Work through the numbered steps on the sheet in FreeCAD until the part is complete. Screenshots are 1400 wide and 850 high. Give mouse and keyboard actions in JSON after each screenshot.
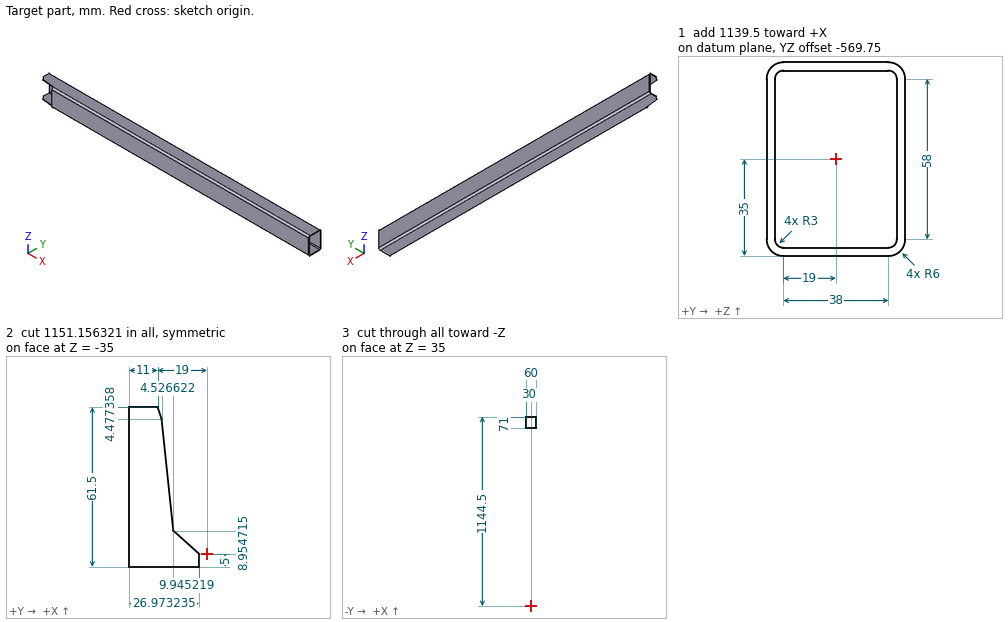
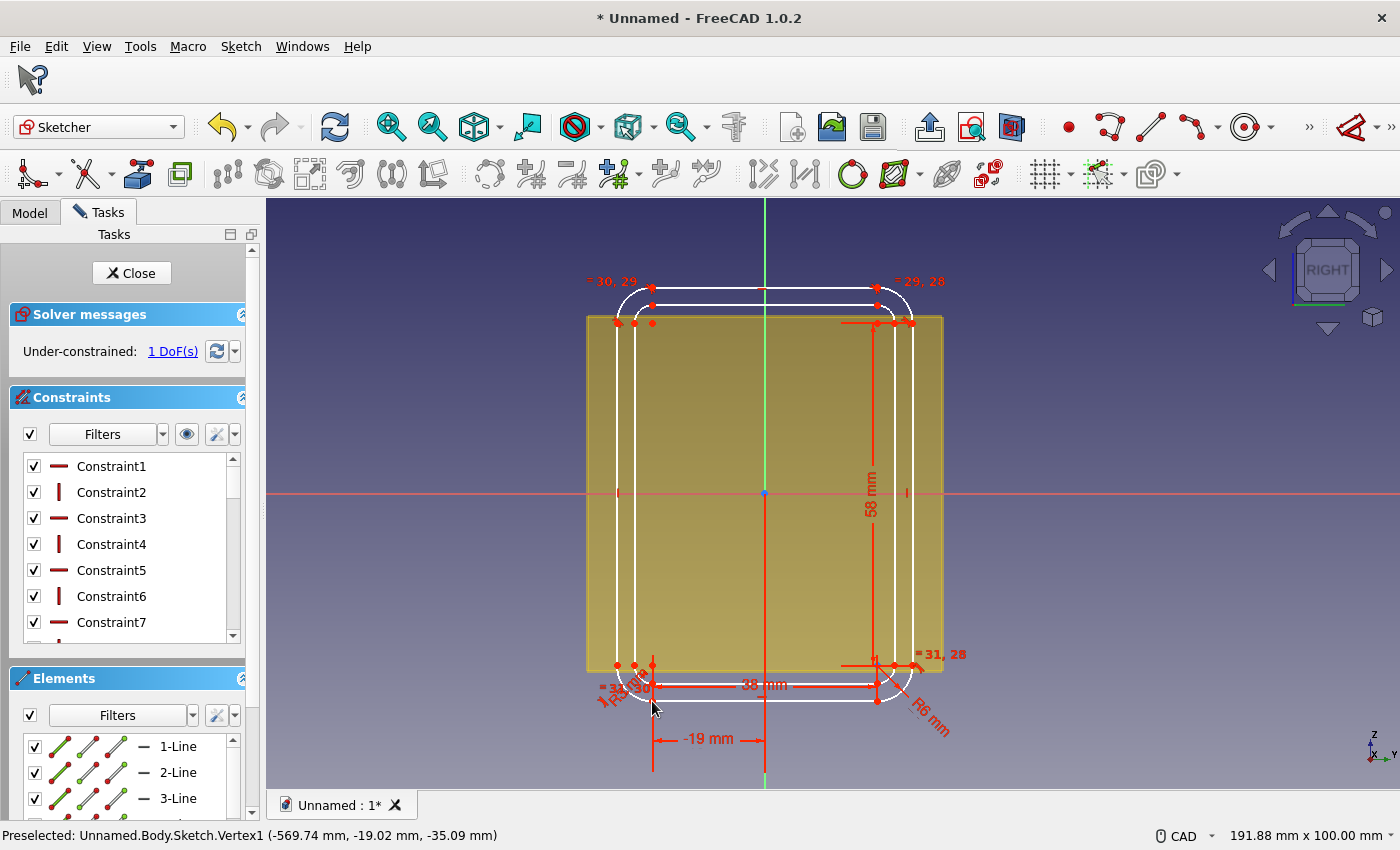
{"action": "left_click", "coordinate": [653, 701]}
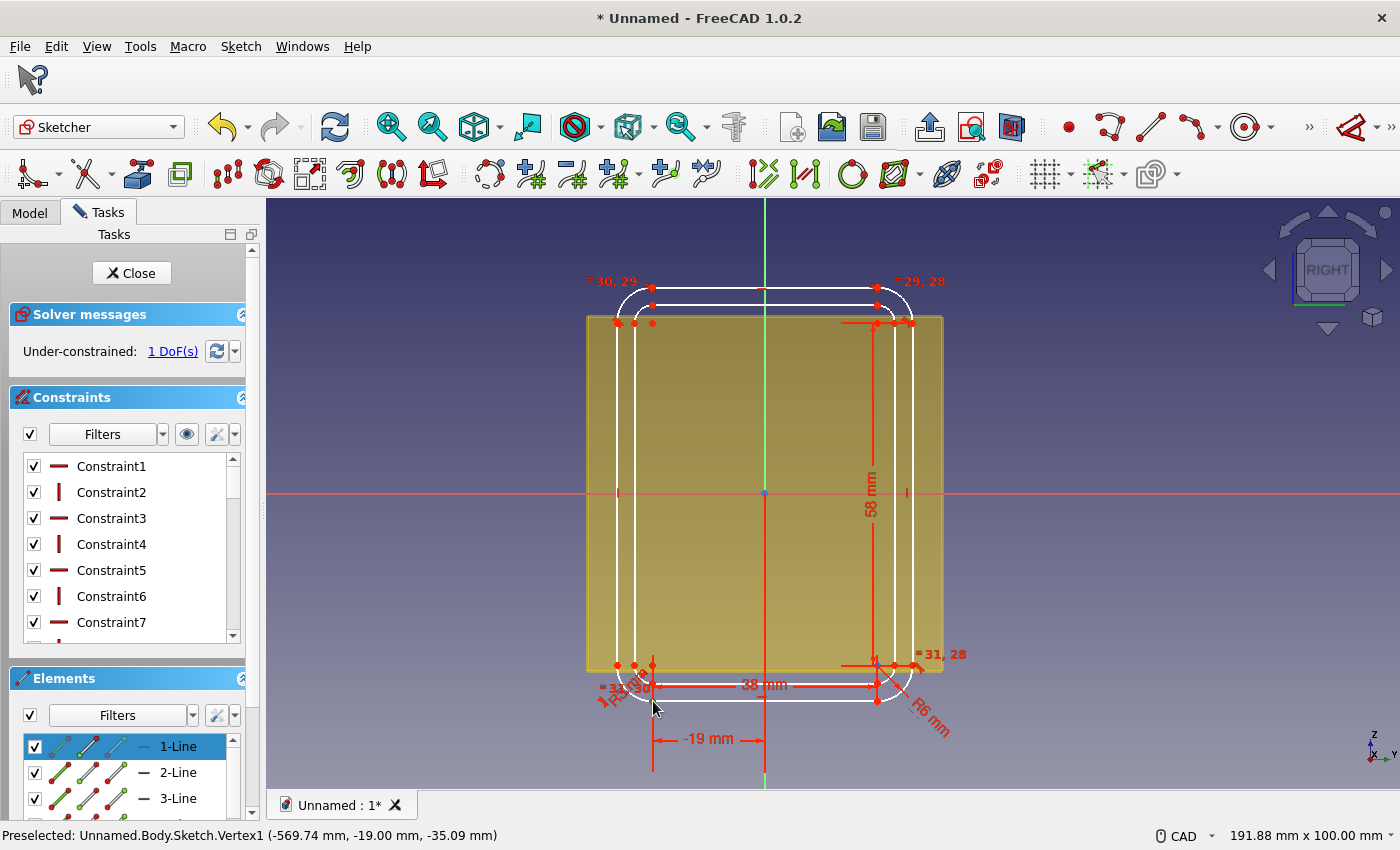
{"action": "left_click", "coordinate": [1376, 128]}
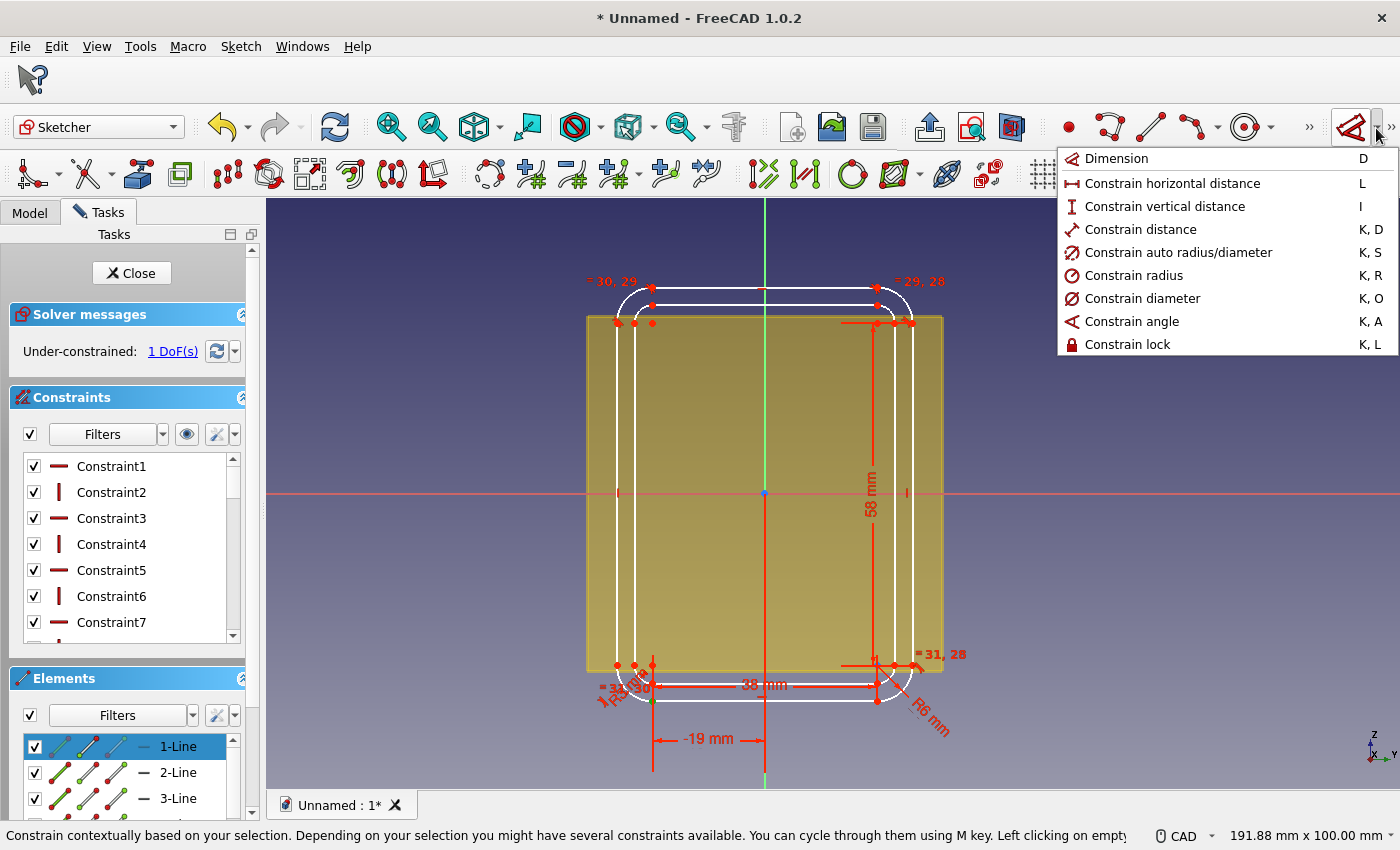
{"action": "left_click", "coordinate": [1228, 206]}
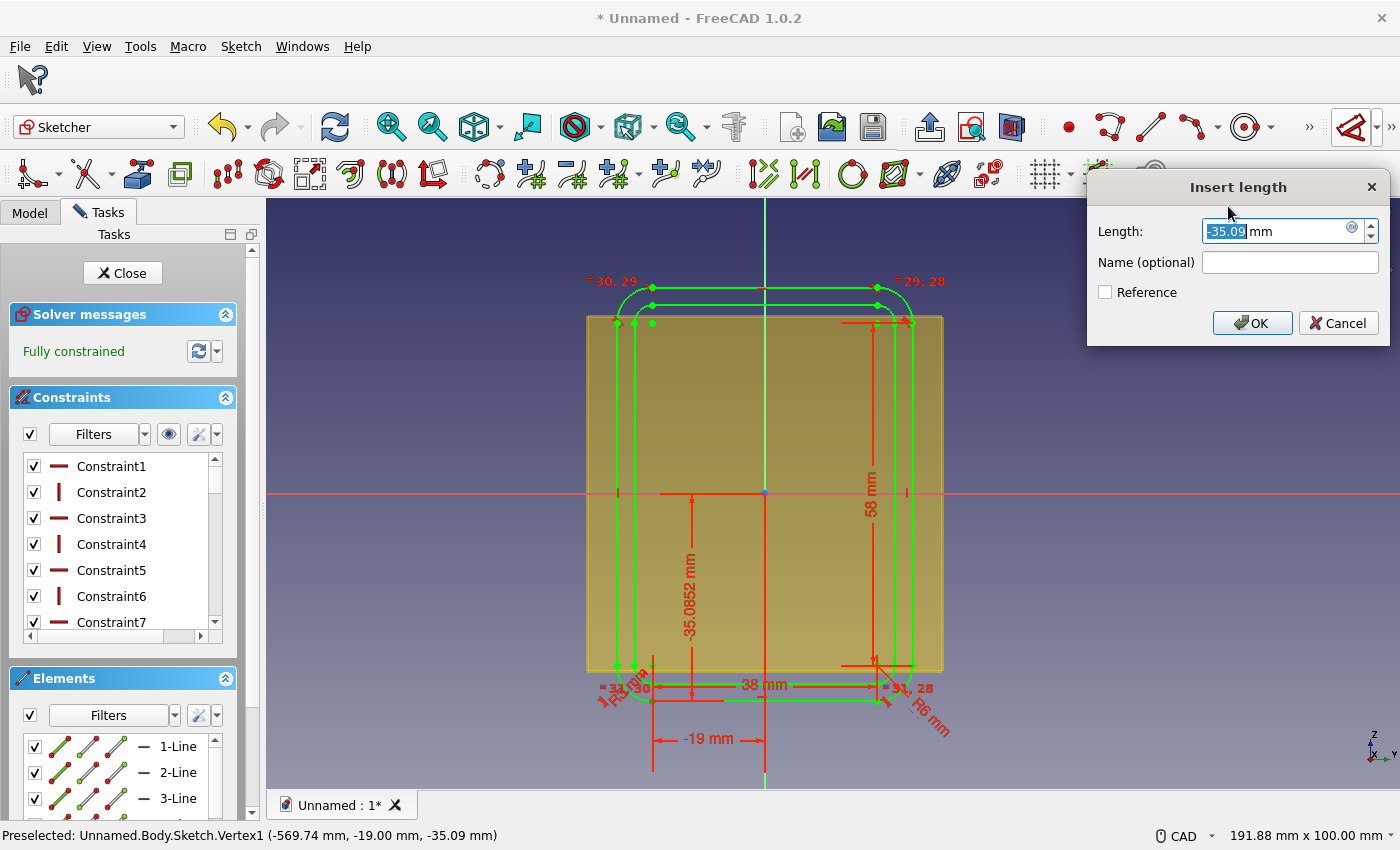
{"action": "type", "text": "-35"}
{"action": "key", "text": "Return"}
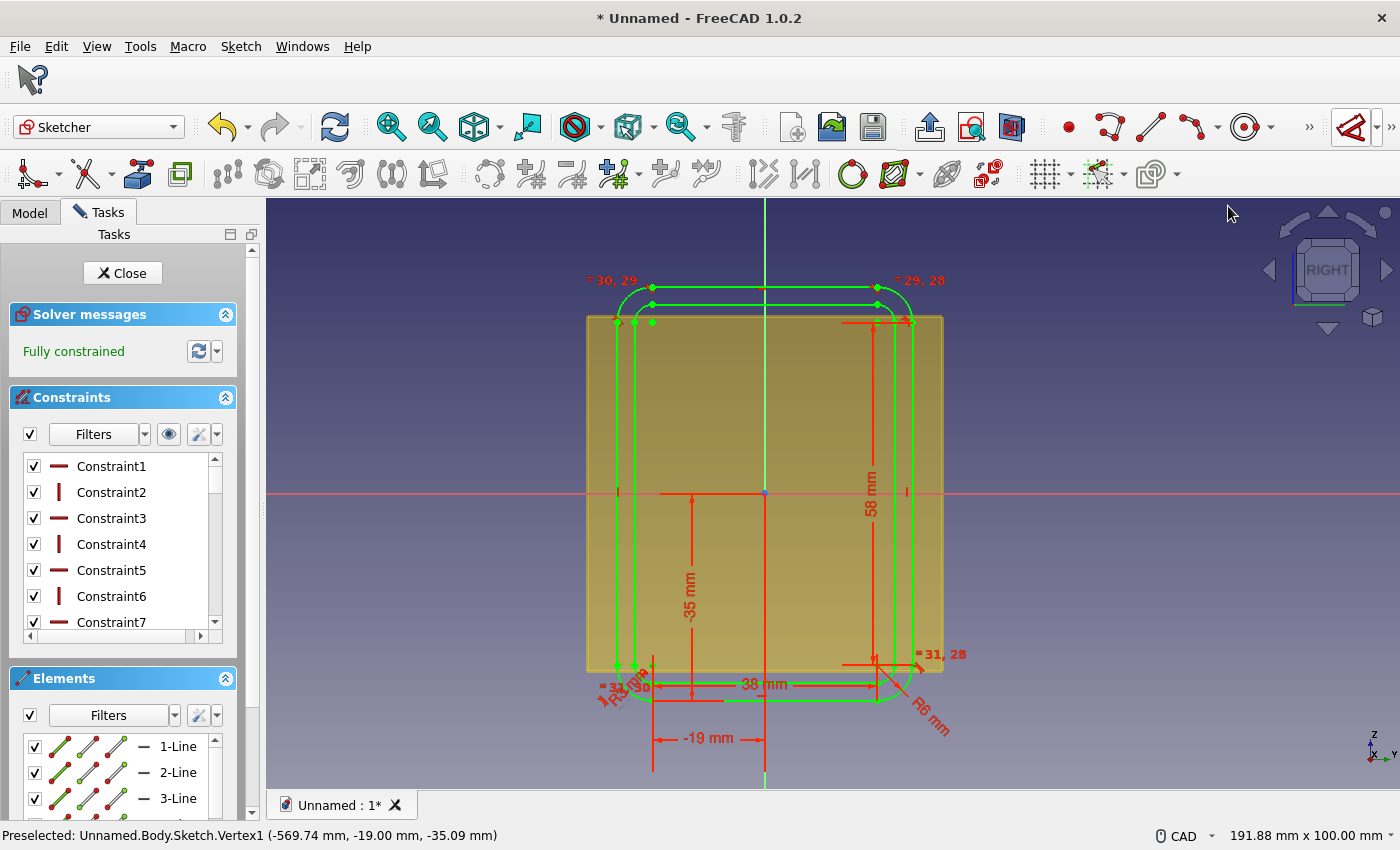
{"action": "left_click", "coordinate": [123, 273]}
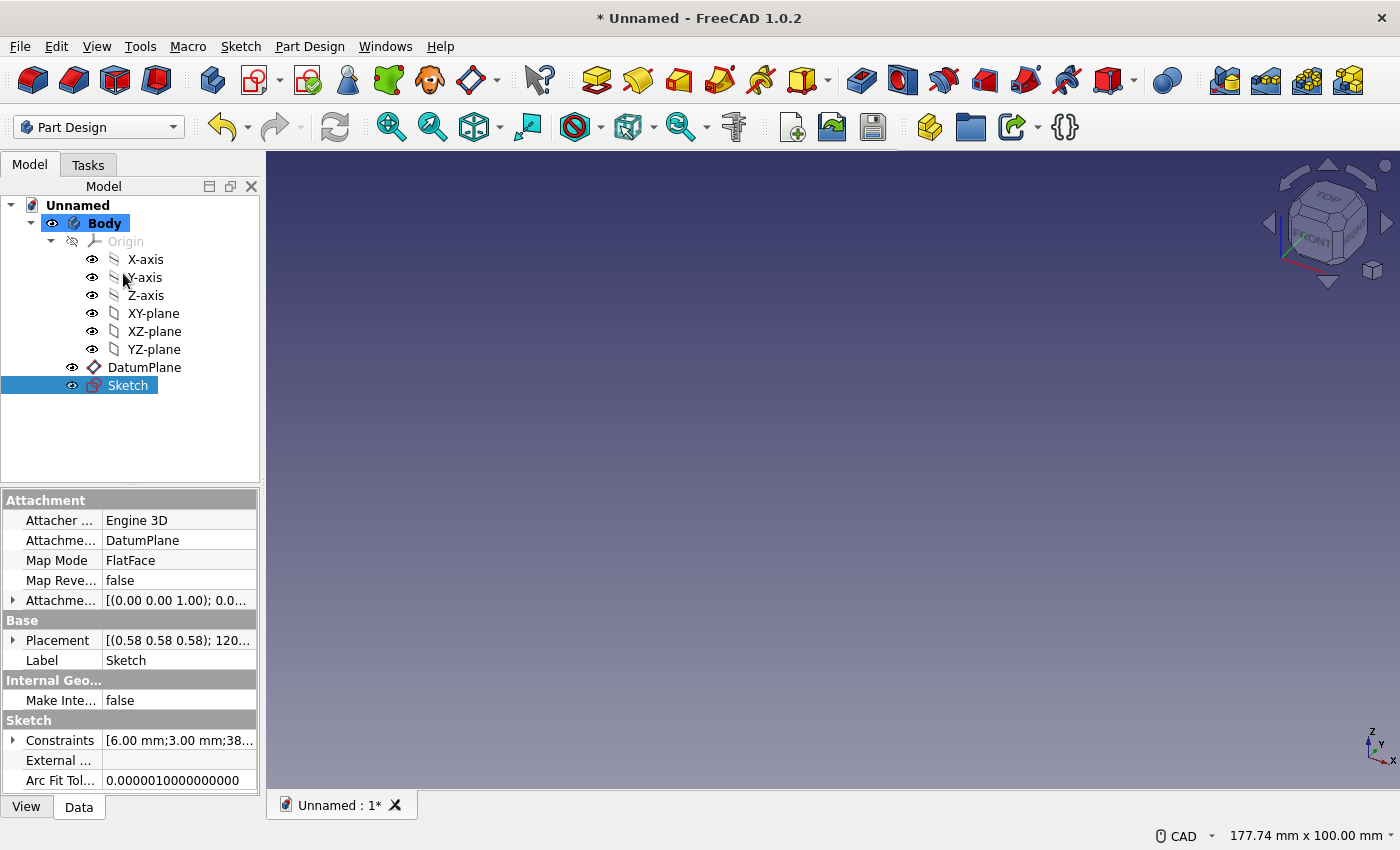
{"action": "left_click", "coordinate": [597, 80]}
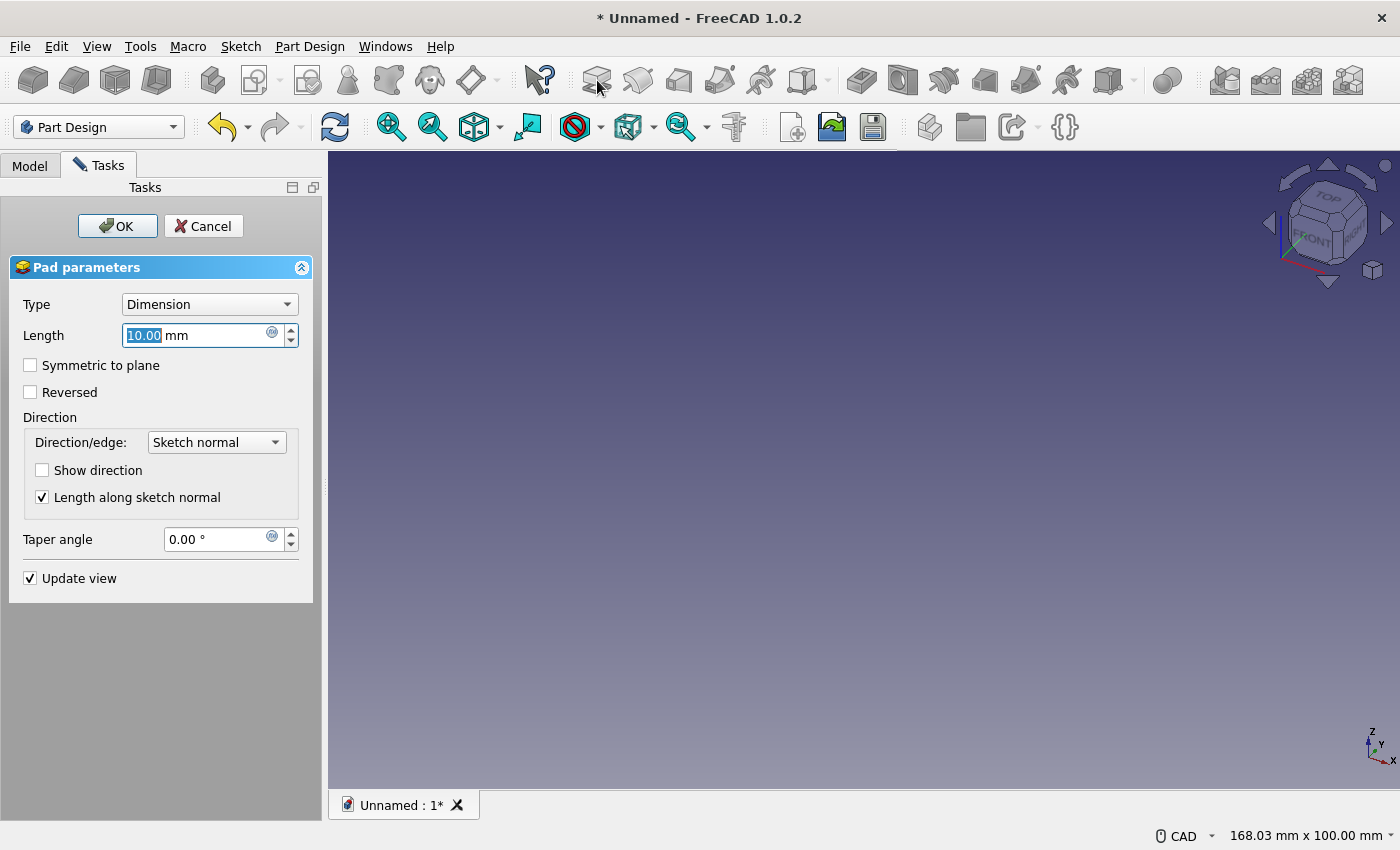
{"action": "type", "text": "1139.5"}
{"action": "key", "text": "Tab"}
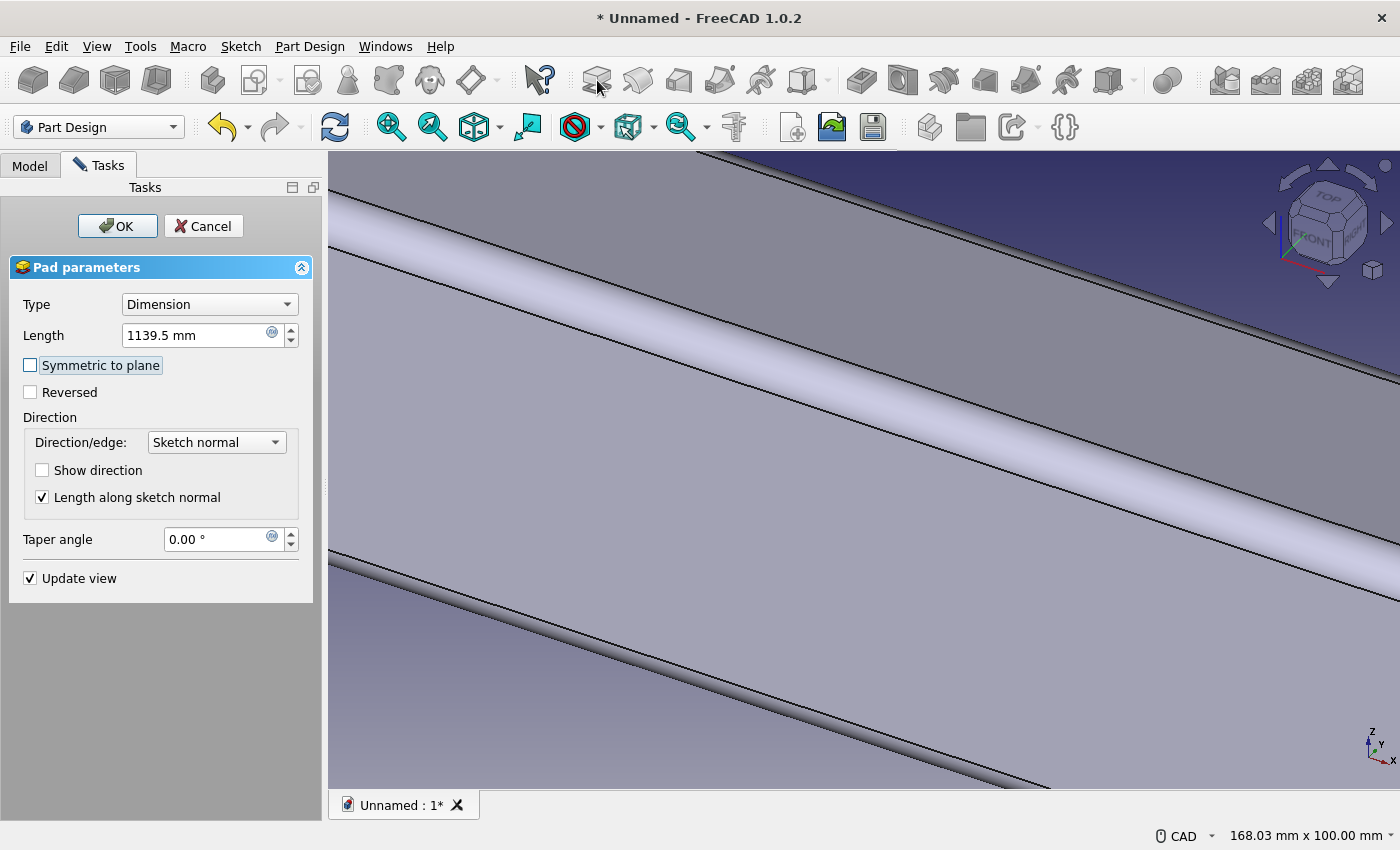
{"action": "left_click", "coordinate": [118, 226]}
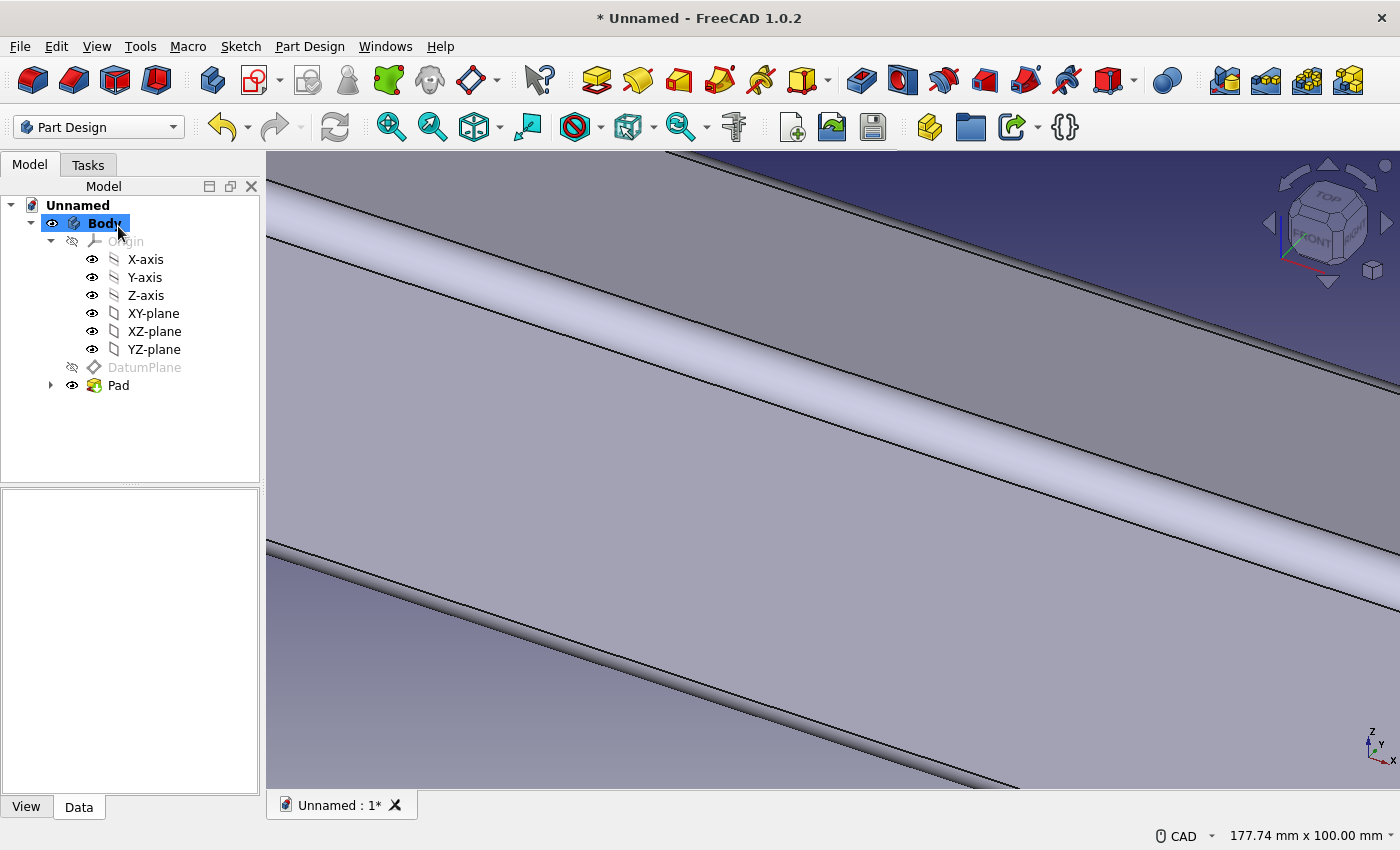
{"action": "key", "text": "v f"}